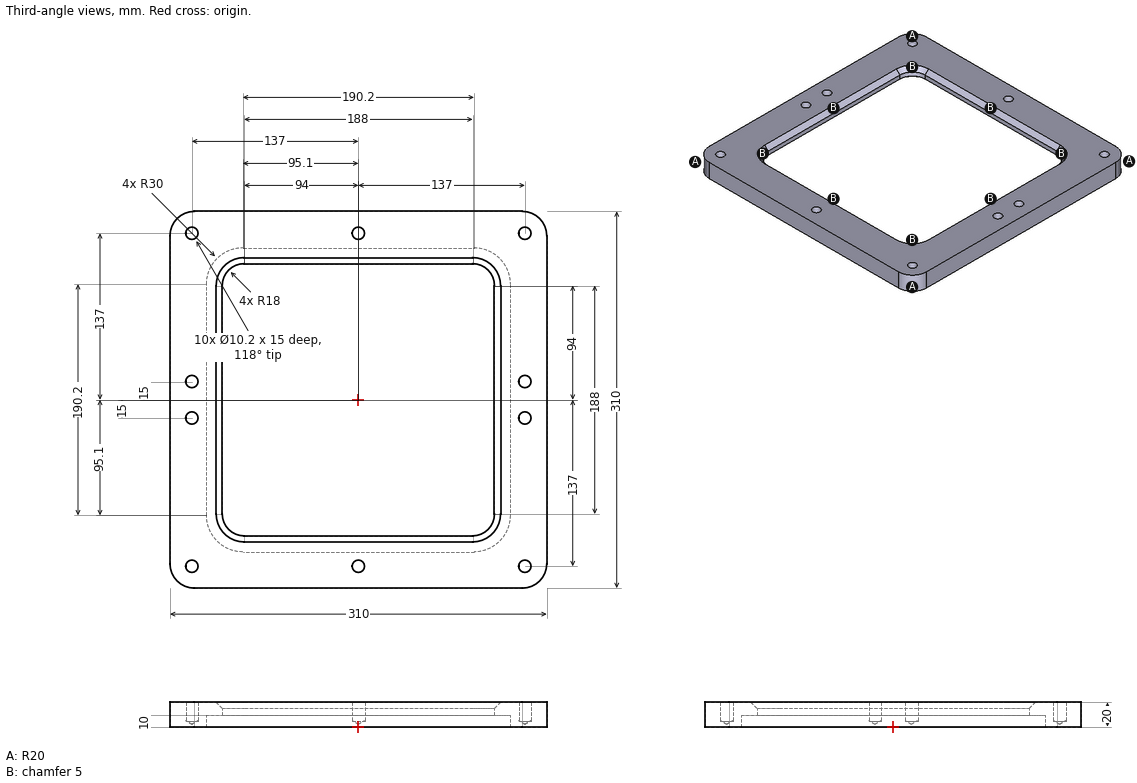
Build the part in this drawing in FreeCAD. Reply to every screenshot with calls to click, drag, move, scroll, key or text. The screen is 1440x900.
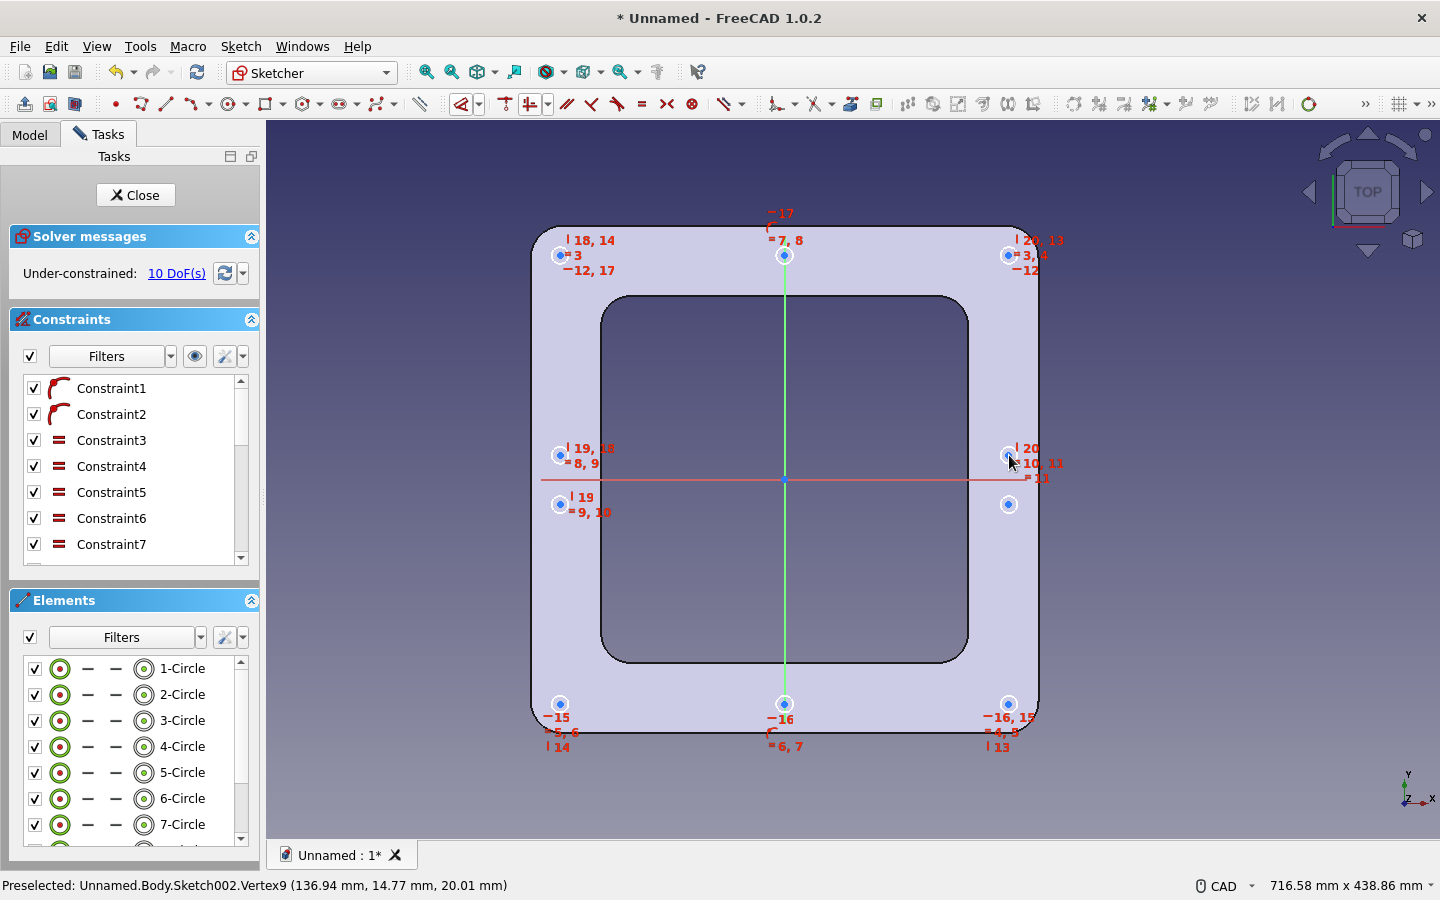
click(560, 455)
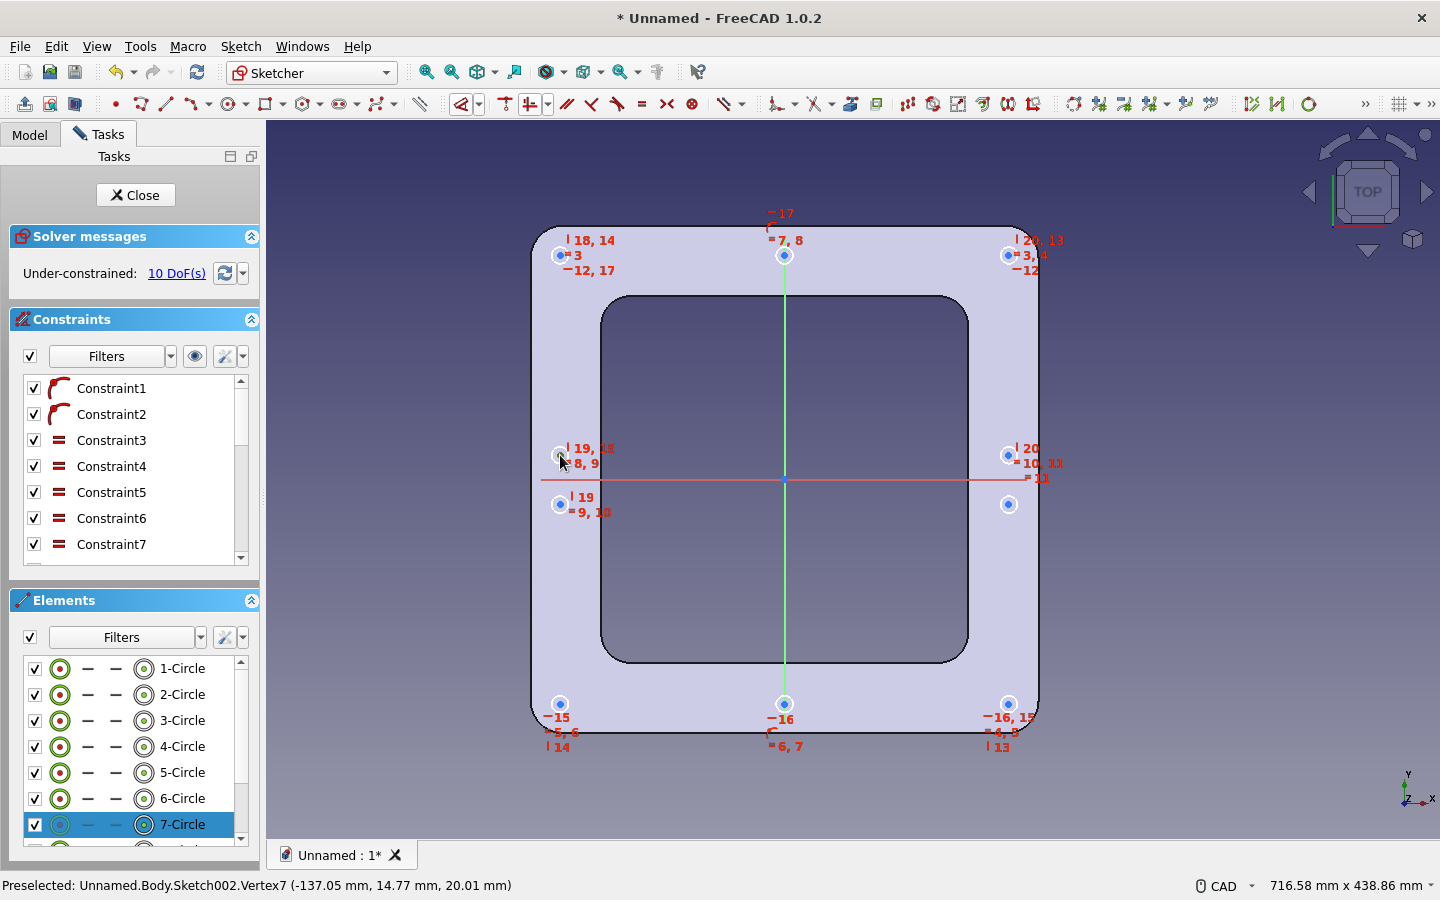
click(1009, 455)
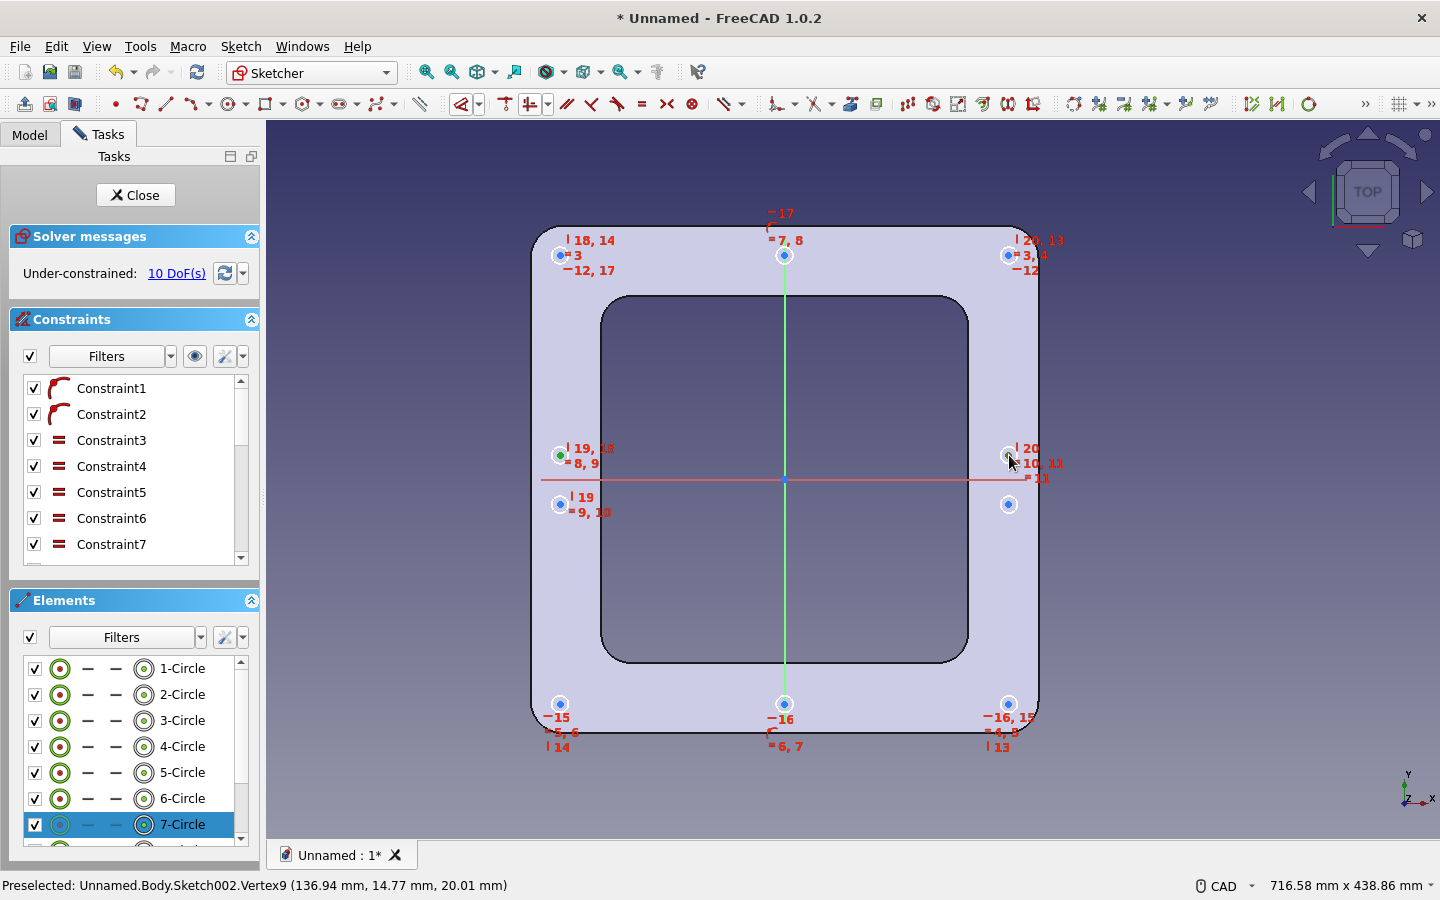
click(548, 104)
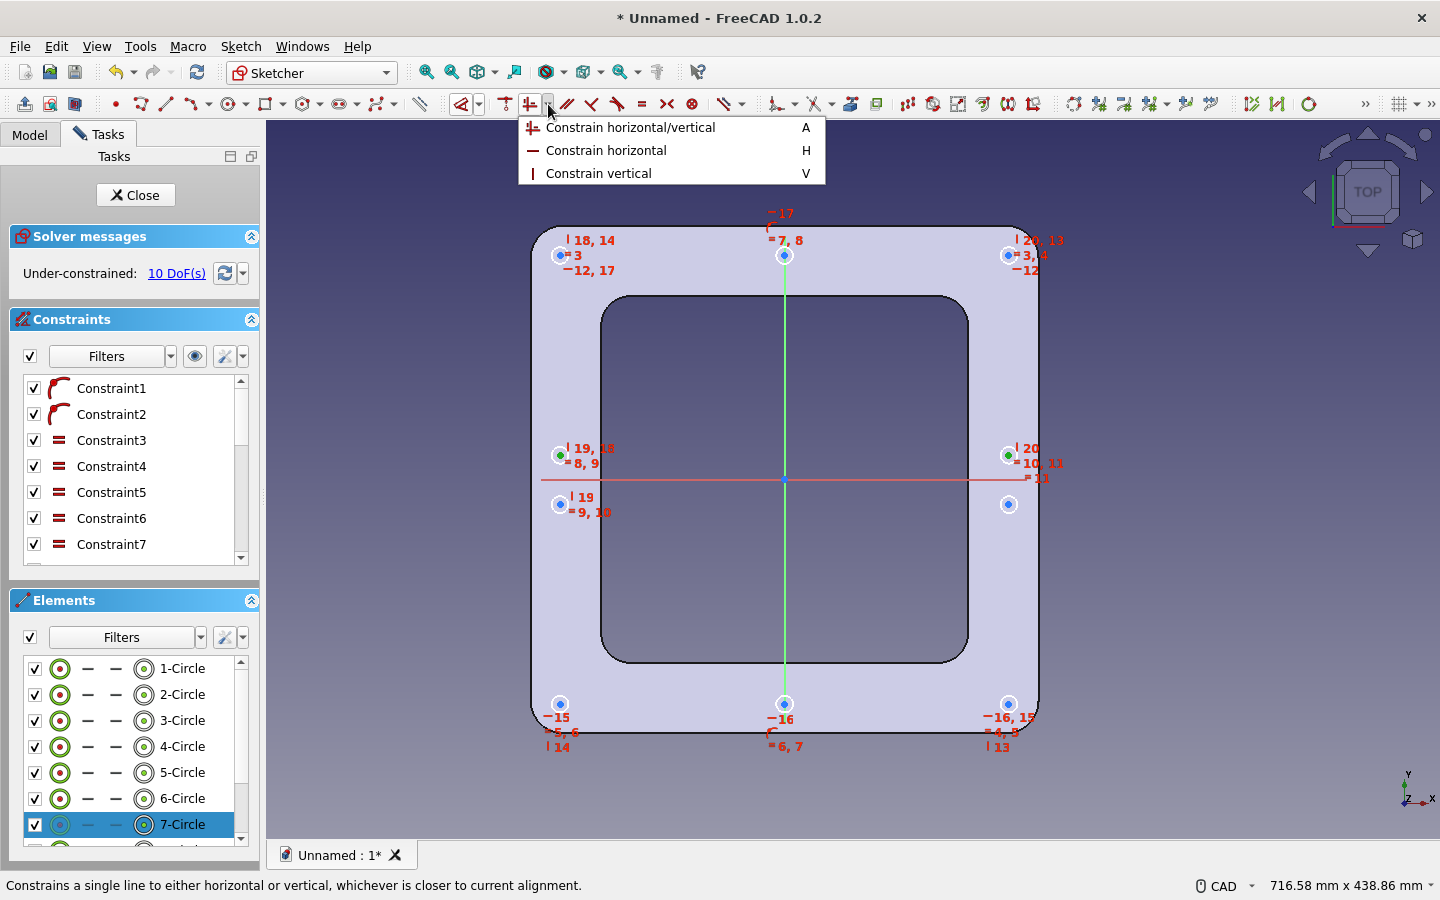
click(672, 150)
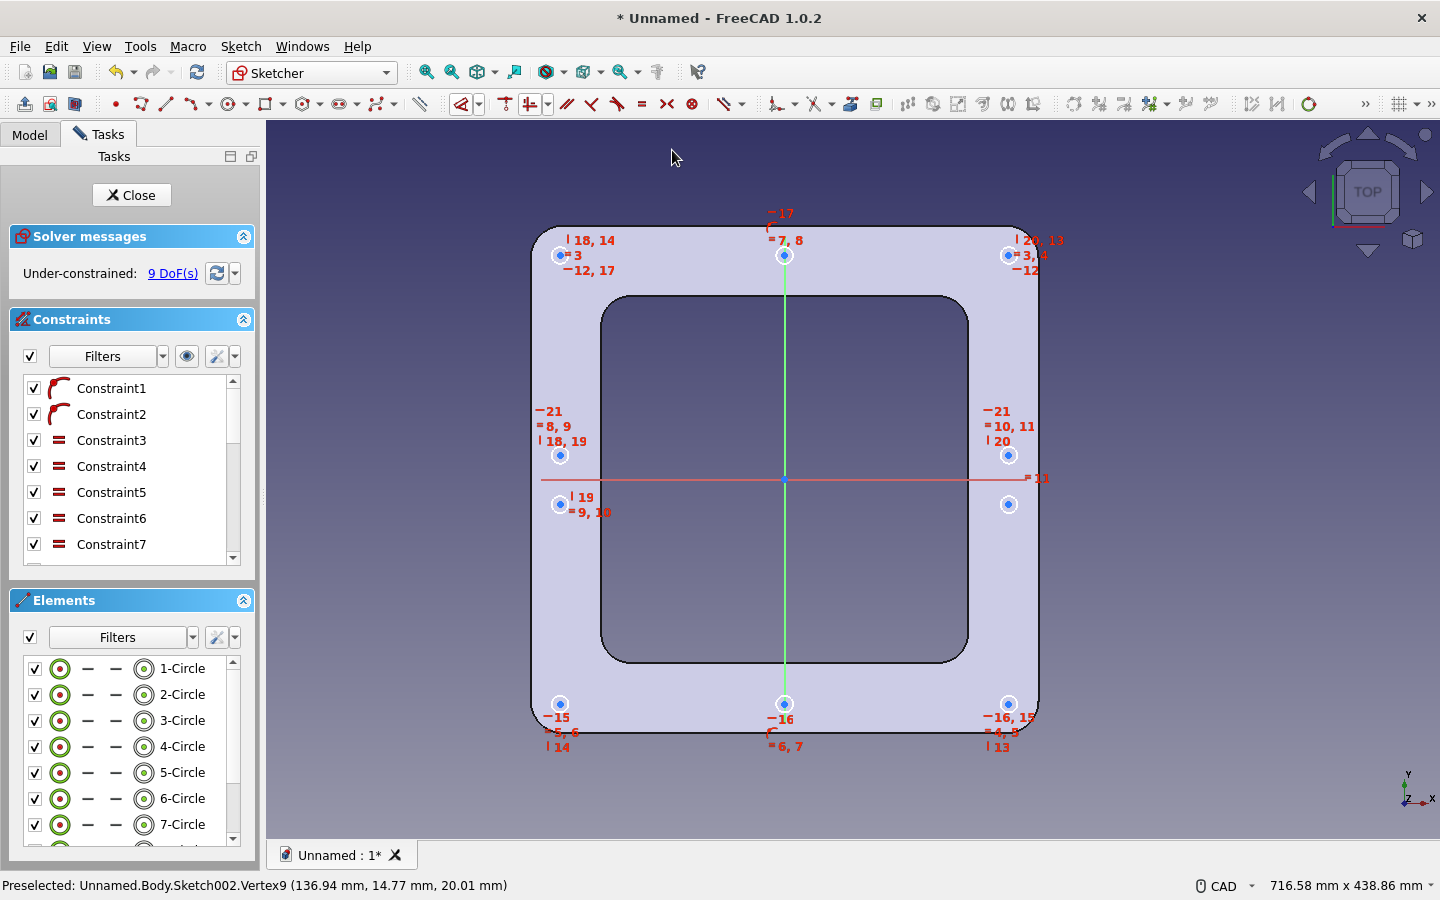
click(1009, 455)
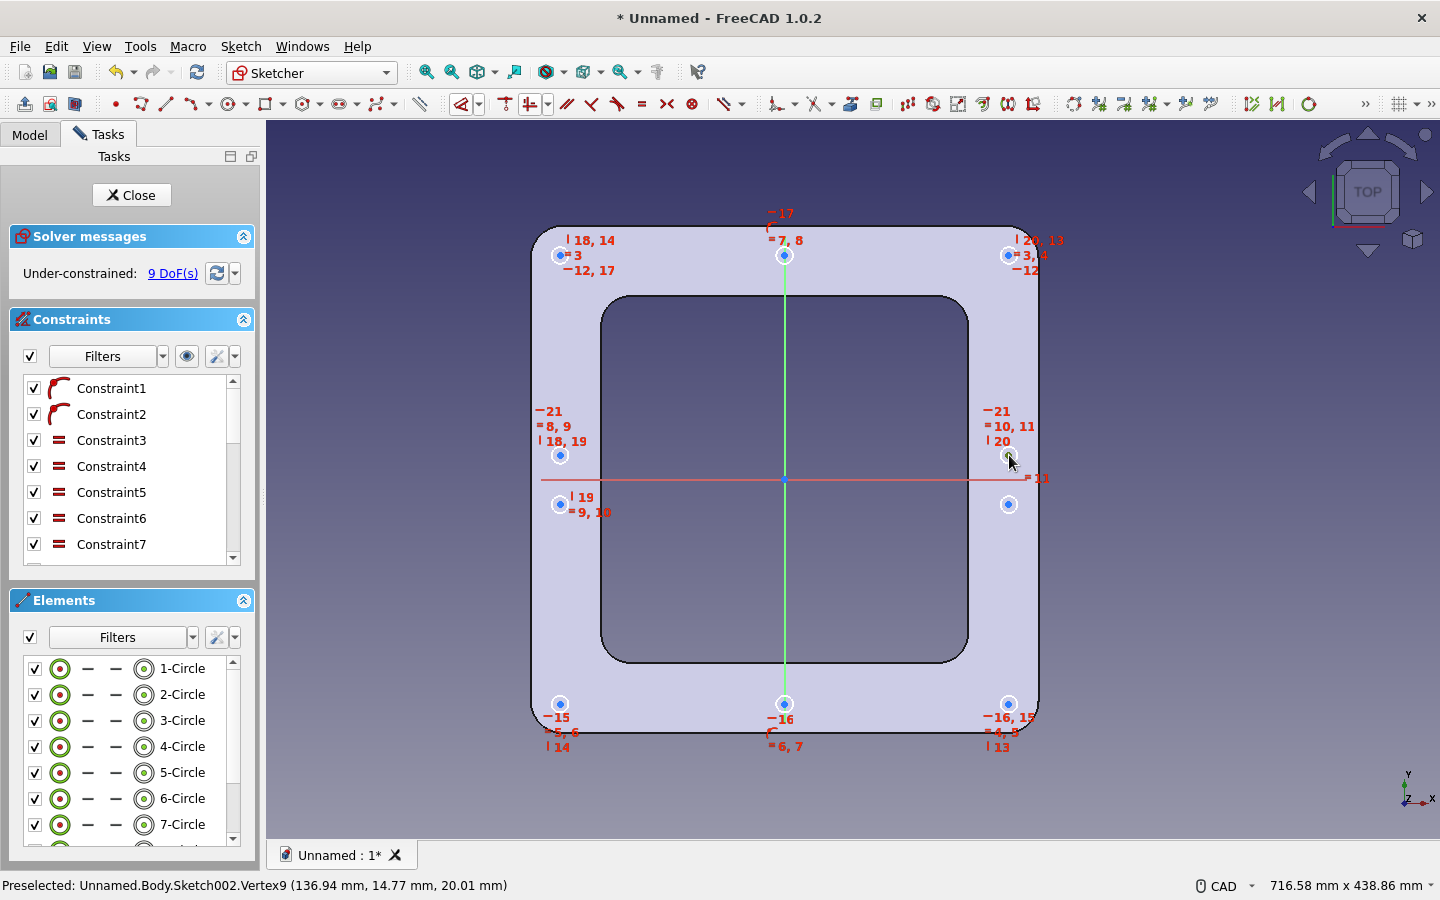
click(1009, 505)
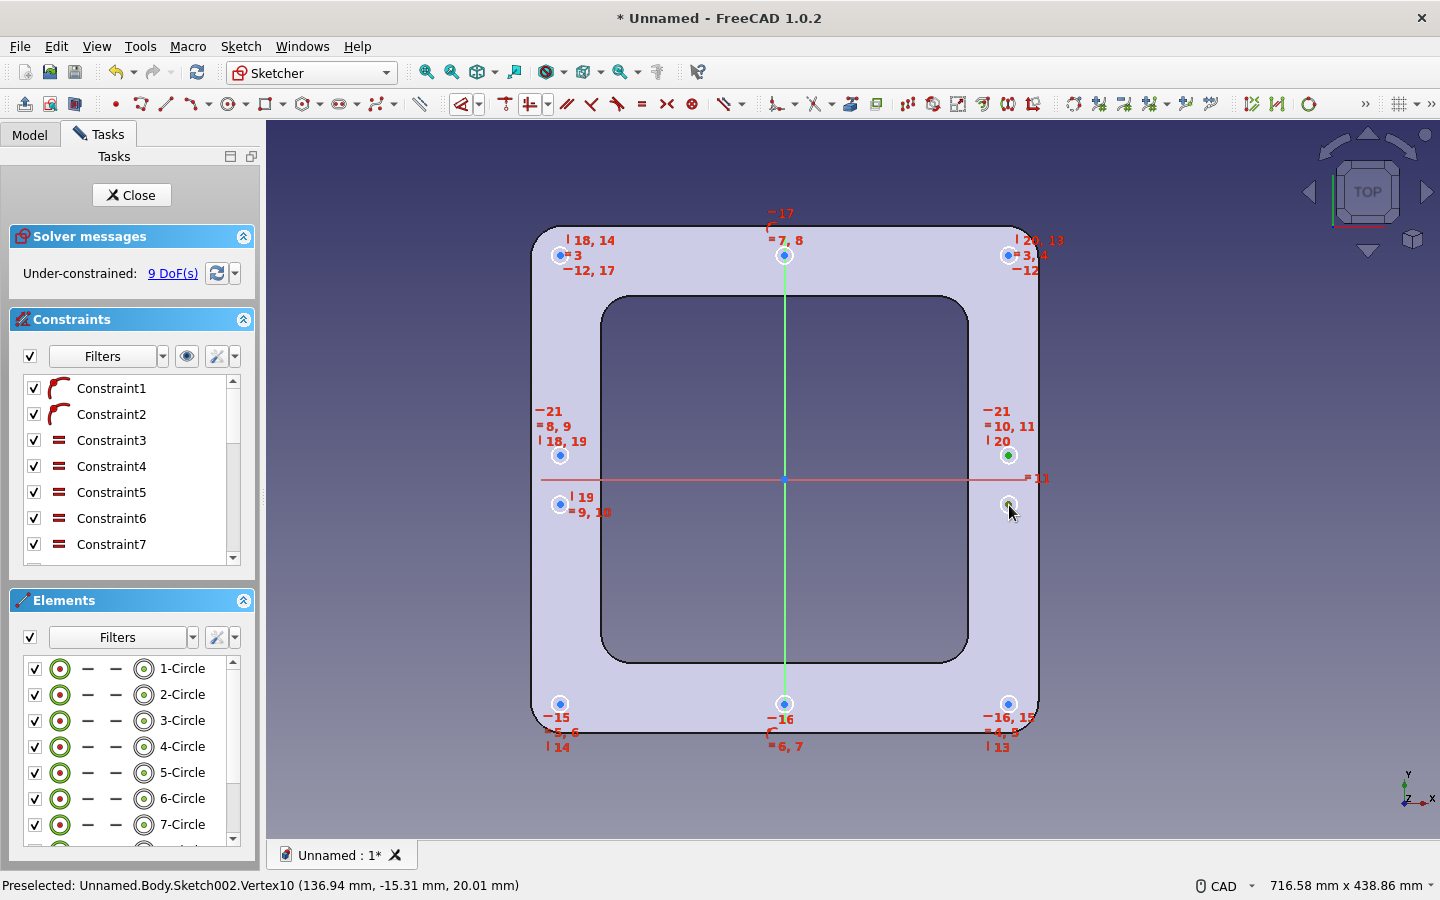
click(548, 104)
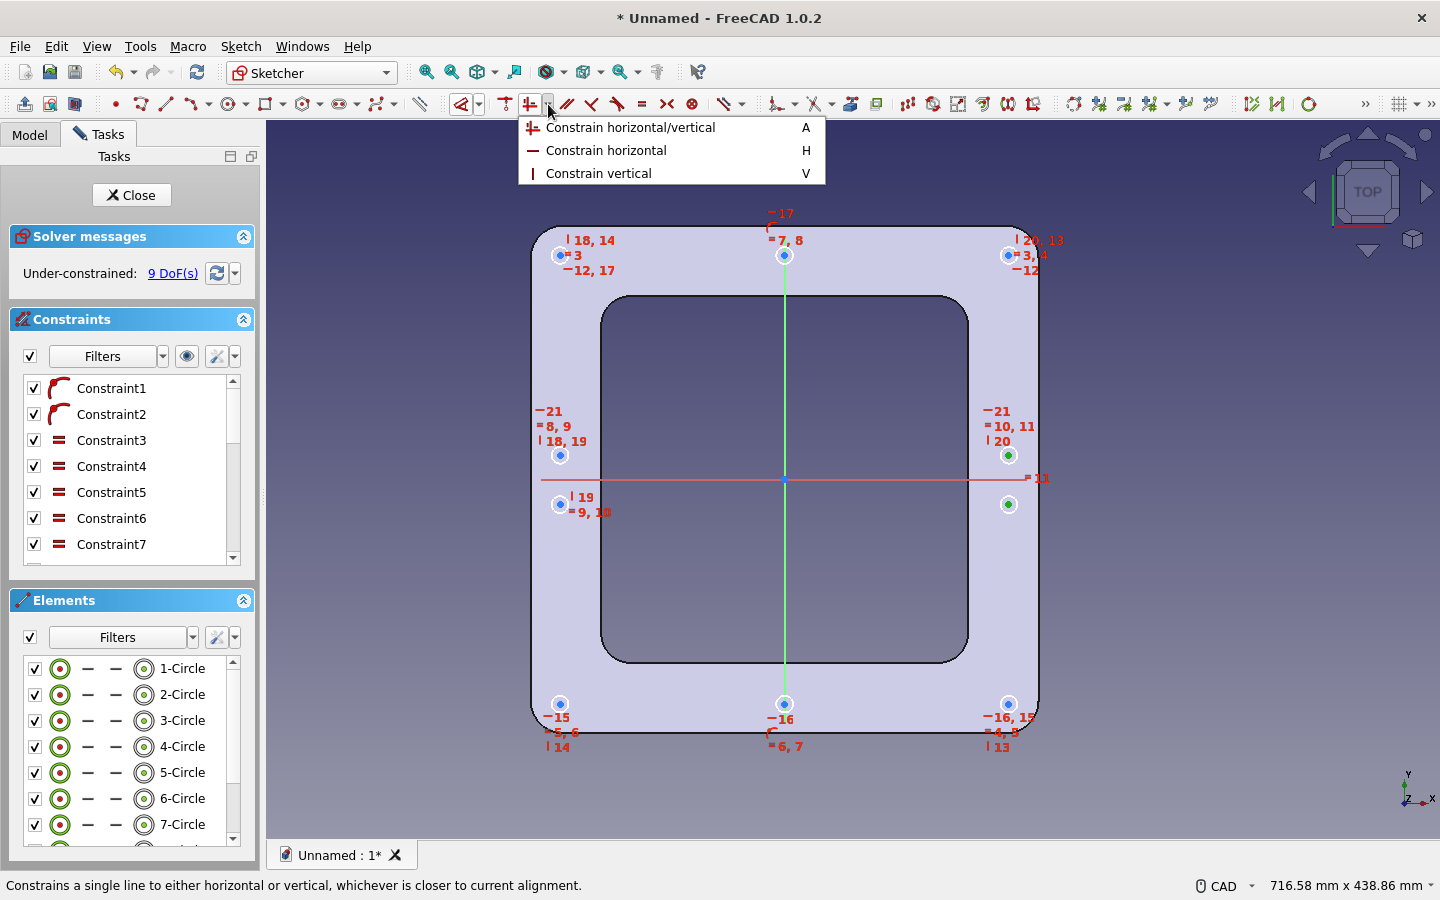
click(672, 174)